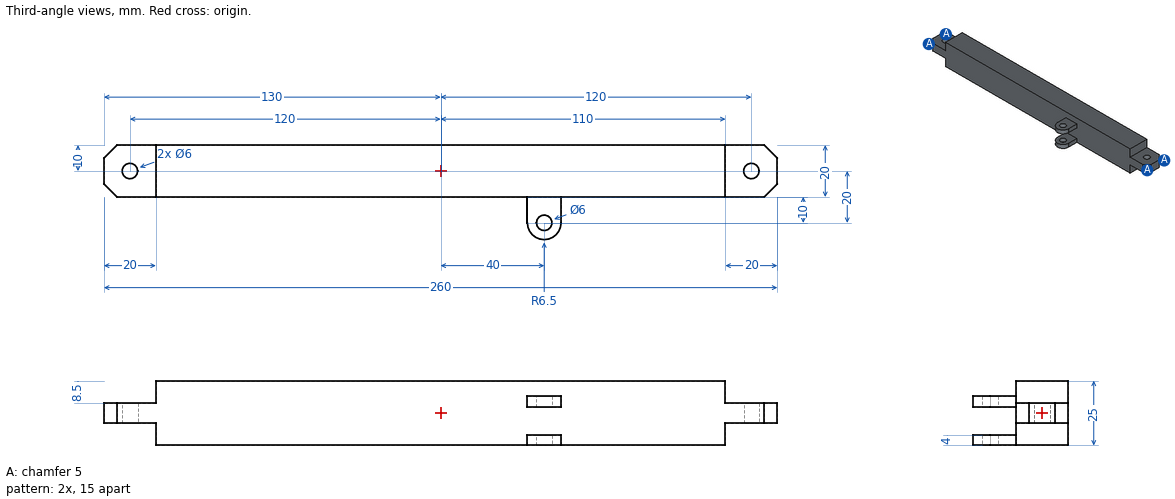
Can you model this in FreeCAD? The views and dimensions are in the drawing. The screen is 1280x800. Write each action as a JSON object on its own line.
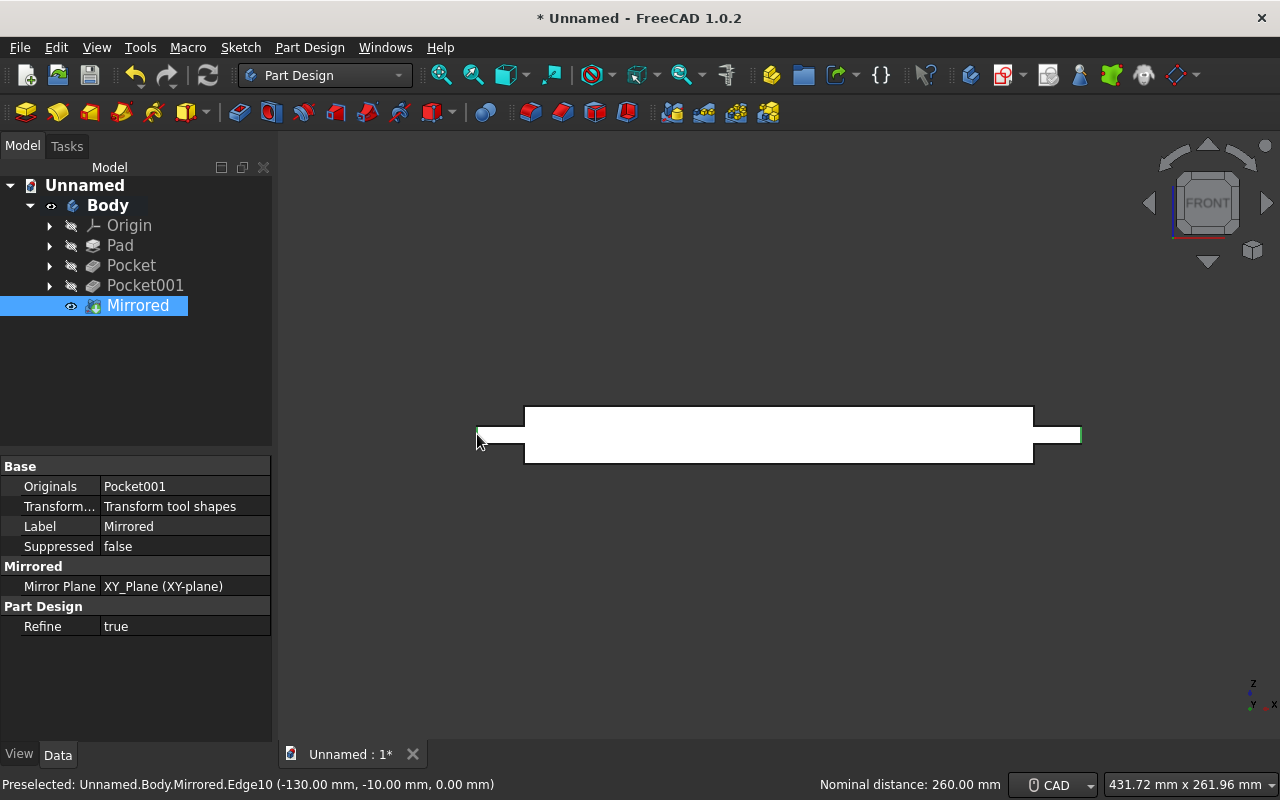
{"action": "scroll", "coordinate": [477, 434], "scroll_direction": "up", "scroll_amount": 4}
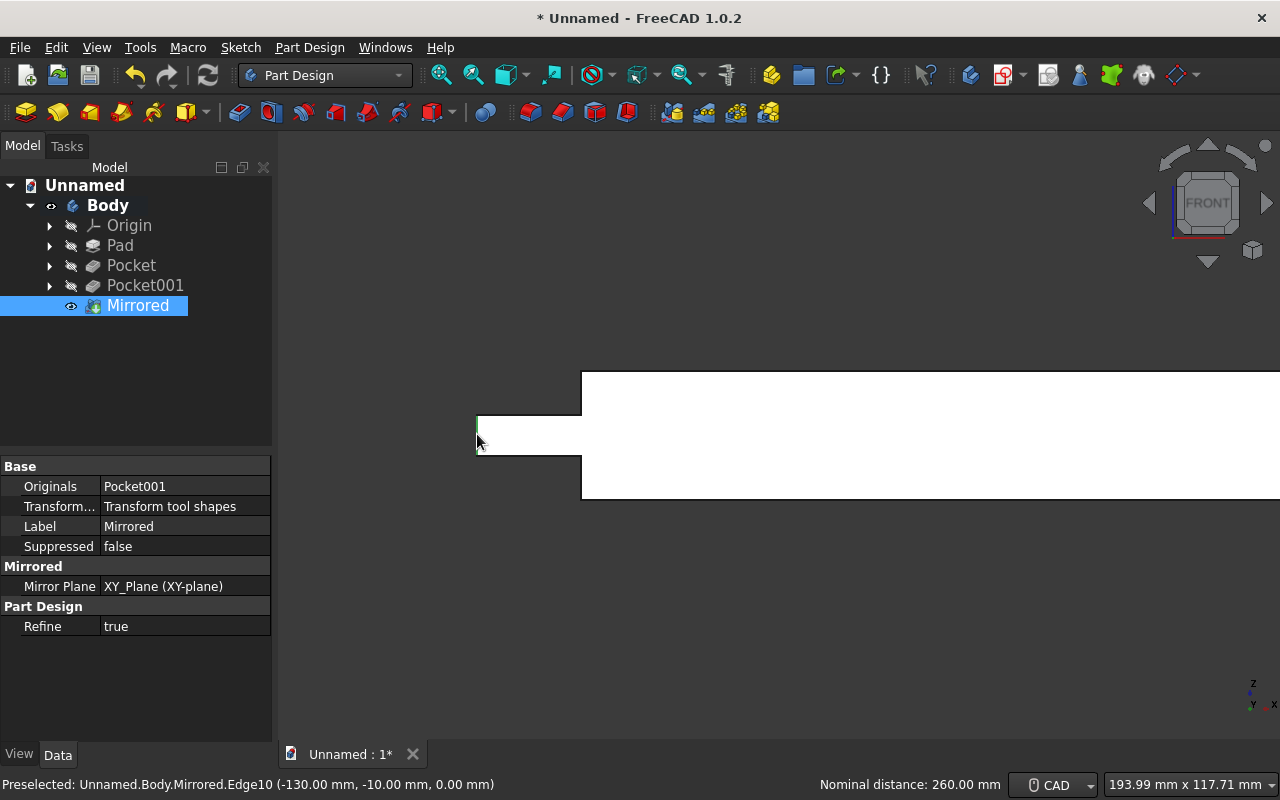
{"action": "left_click", "coordinate": [442, 76]}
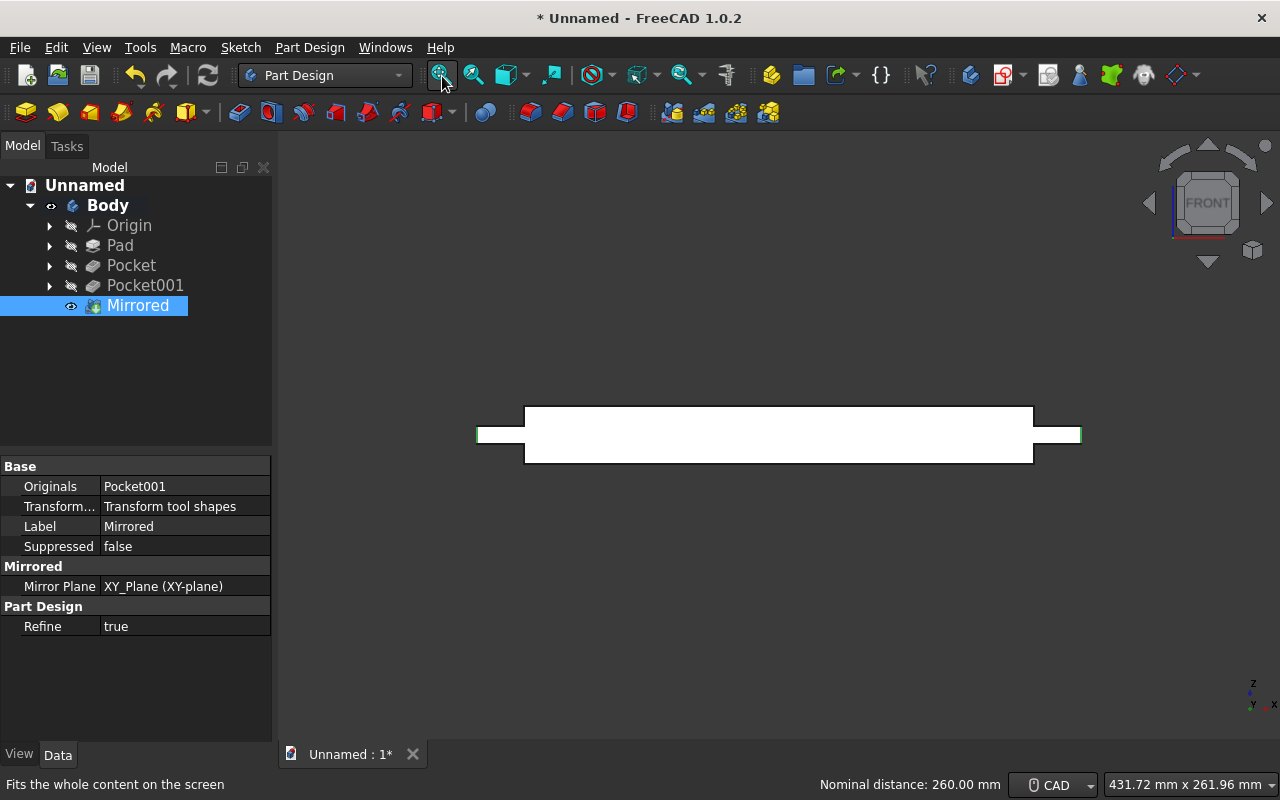
{"action": "key", "text": "3"}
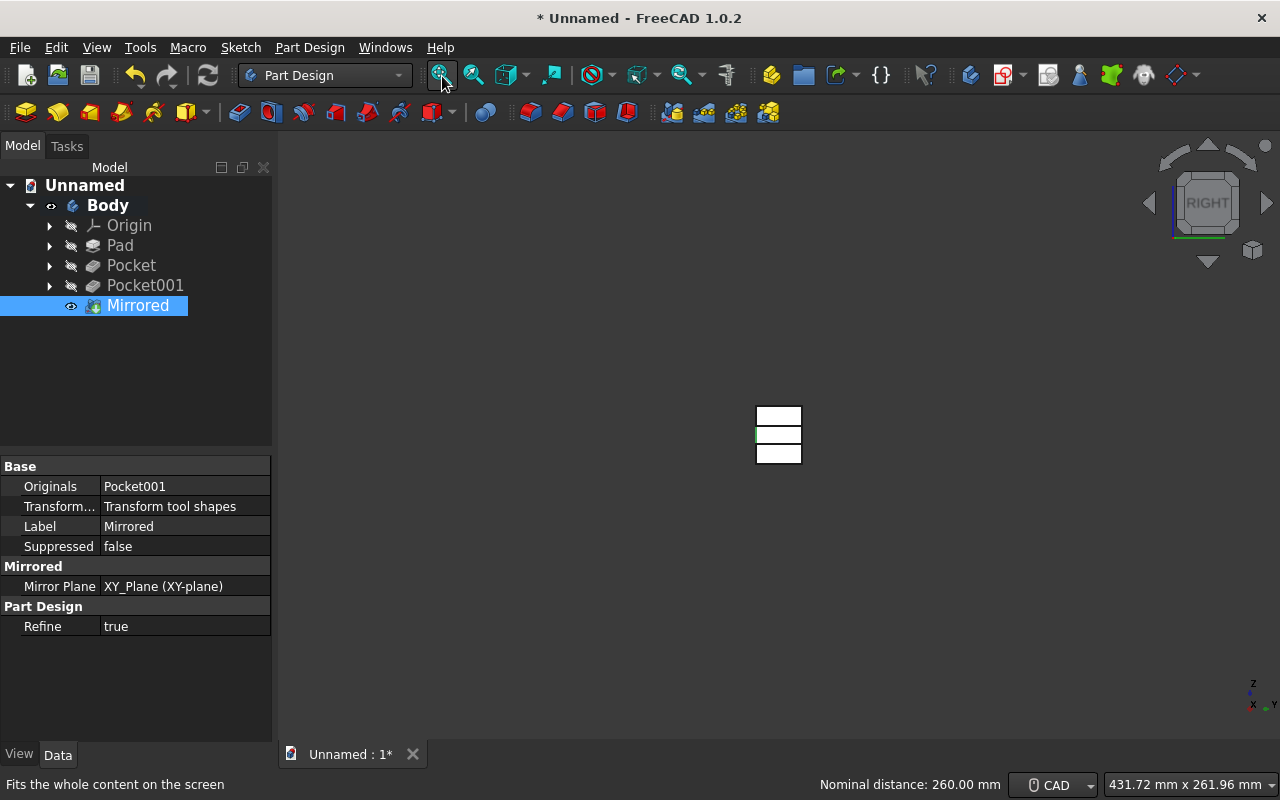
{"action": "key", "text": "v f"}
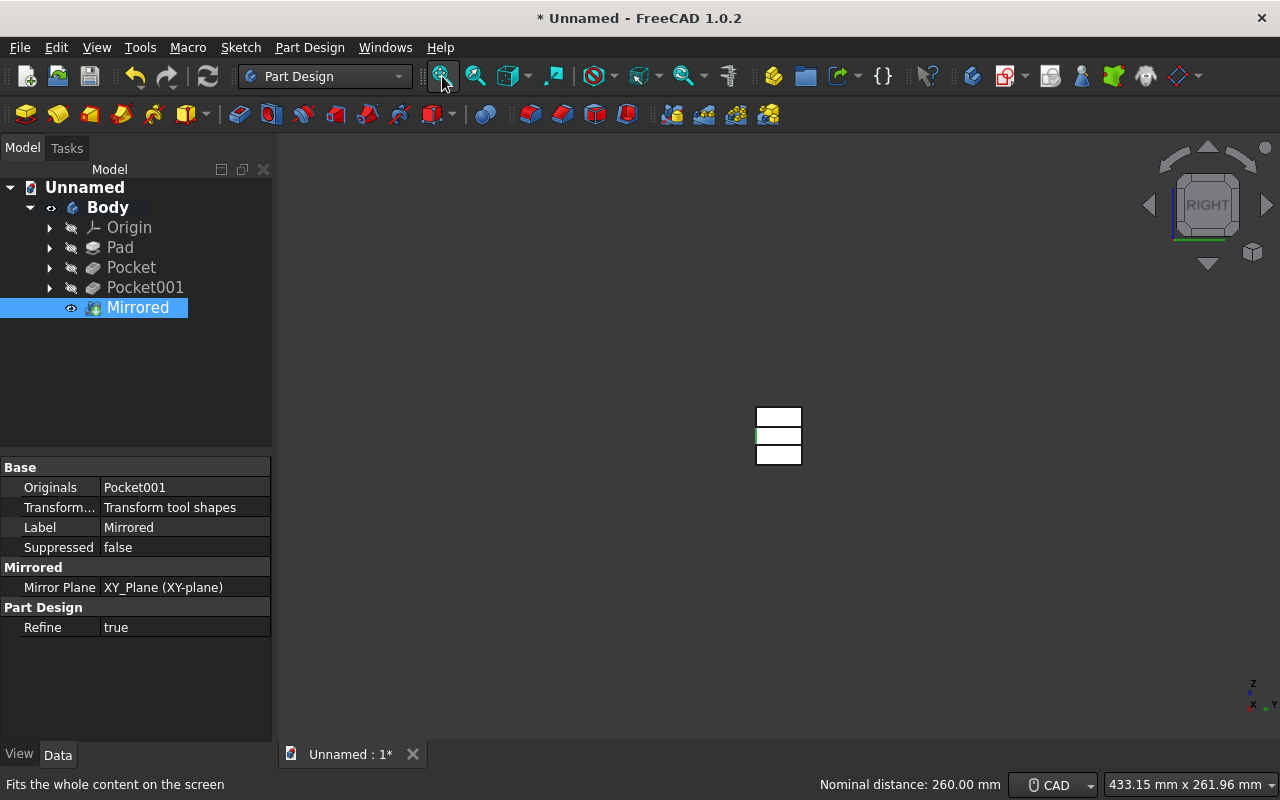
{"action": "left_click", "coordinate": [802, 435], "text": "ctrl"}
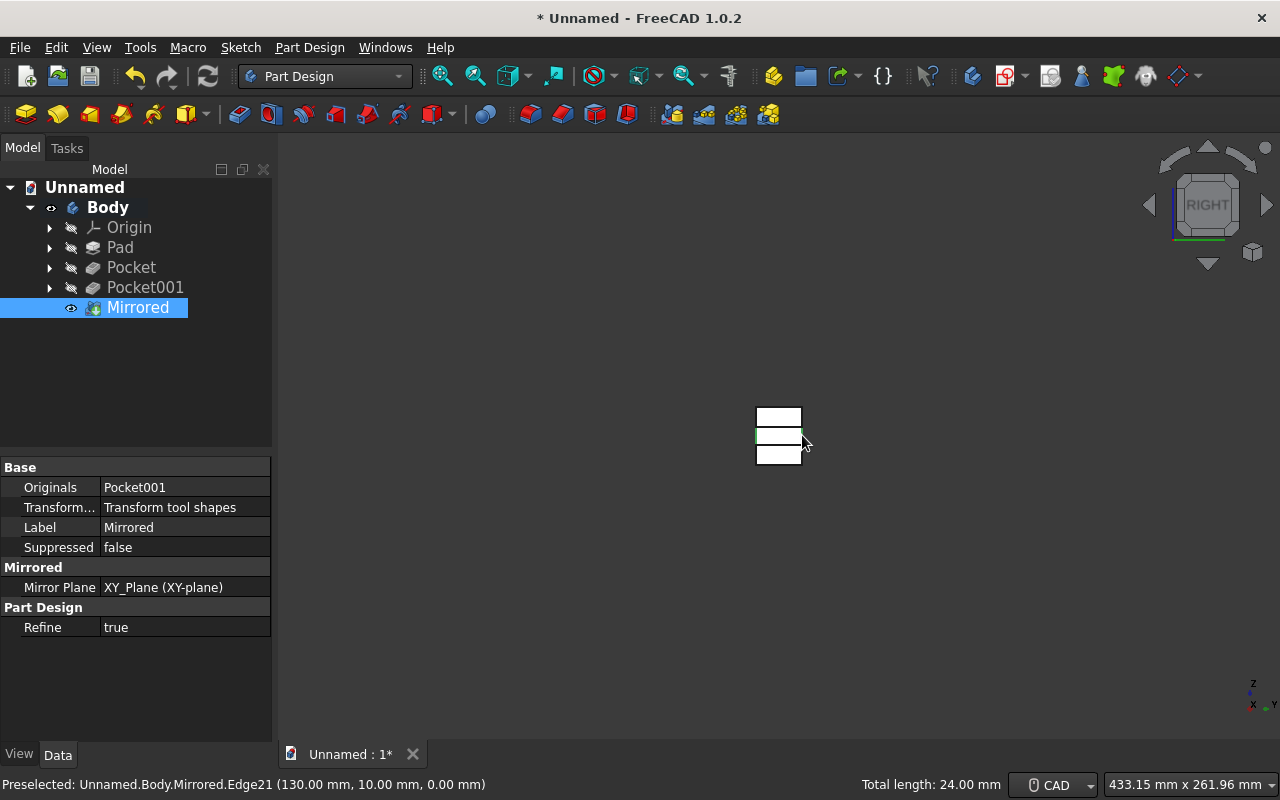
{"action": "scroll", "coordinate": [802, 435], "scroll_direction": "up", "scroll_amount": 4}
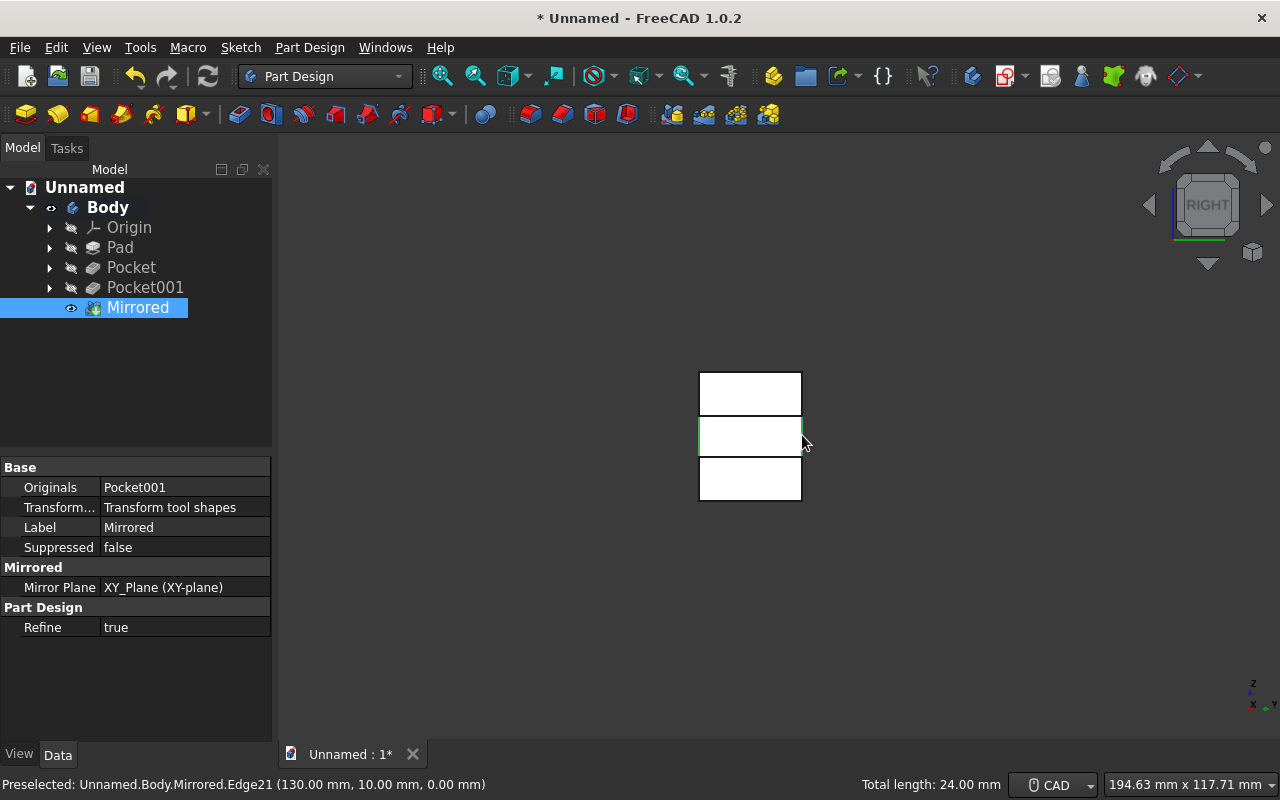
{"action": "key", "text": "v f"}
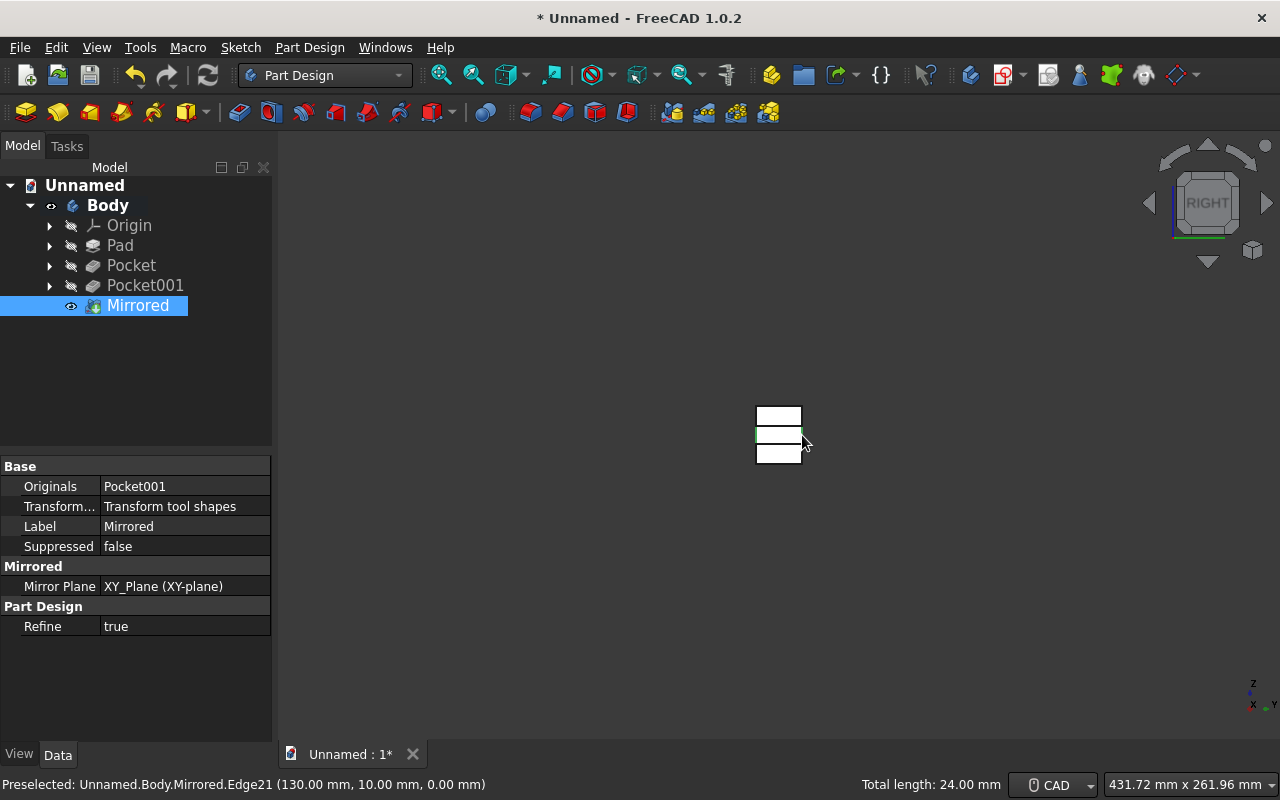
{"action": "key", "text": "5"}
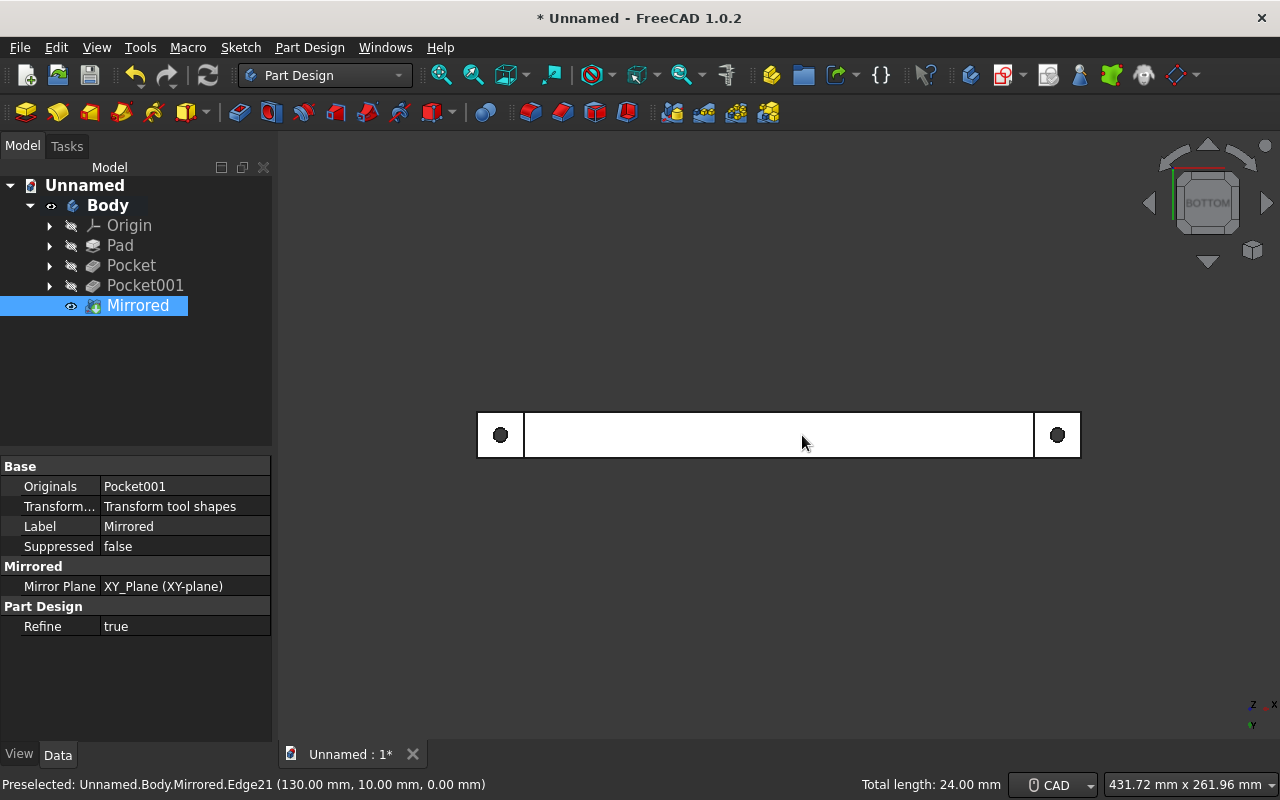
{"action": "scroll", "coordinate": [477, 457], "scroll_direction": "up", "scroll_amount": 4}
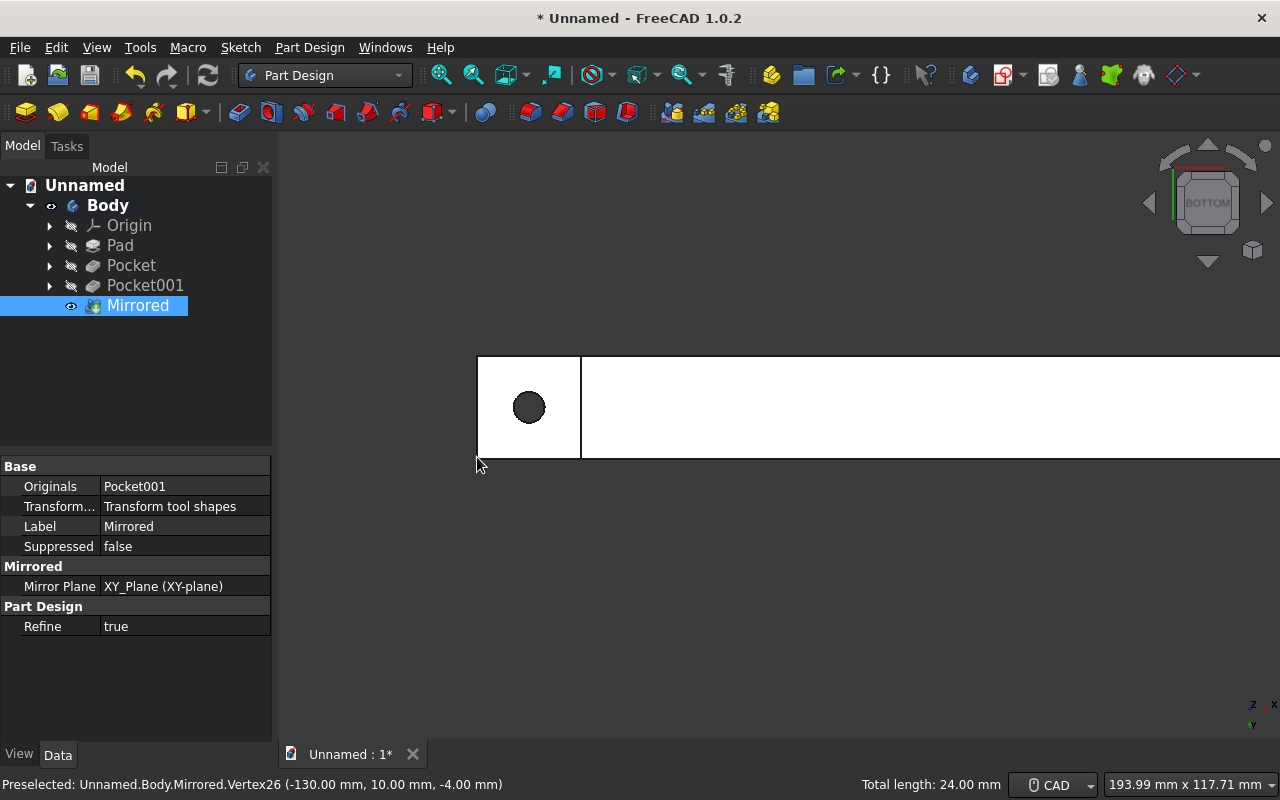
{"action": "key", "text": "v f"}